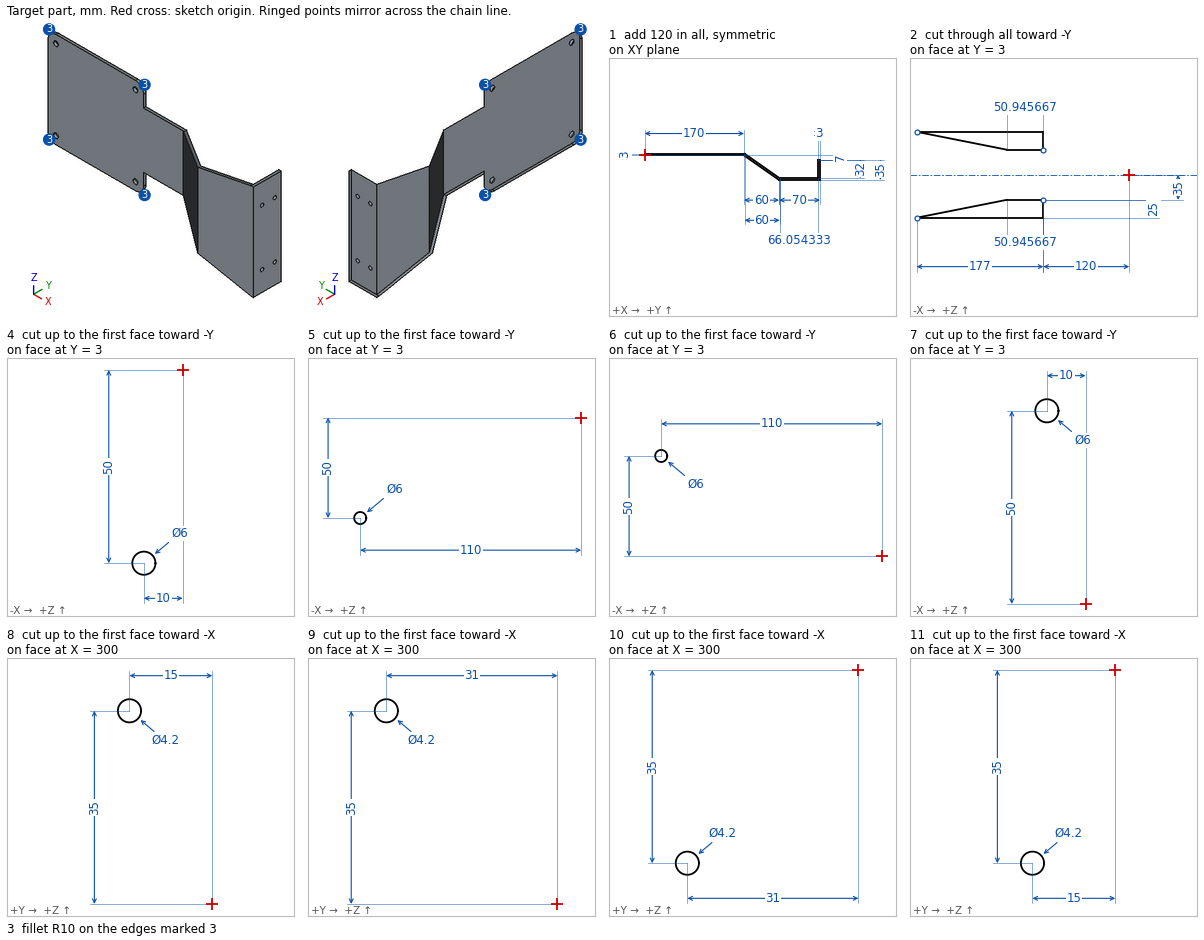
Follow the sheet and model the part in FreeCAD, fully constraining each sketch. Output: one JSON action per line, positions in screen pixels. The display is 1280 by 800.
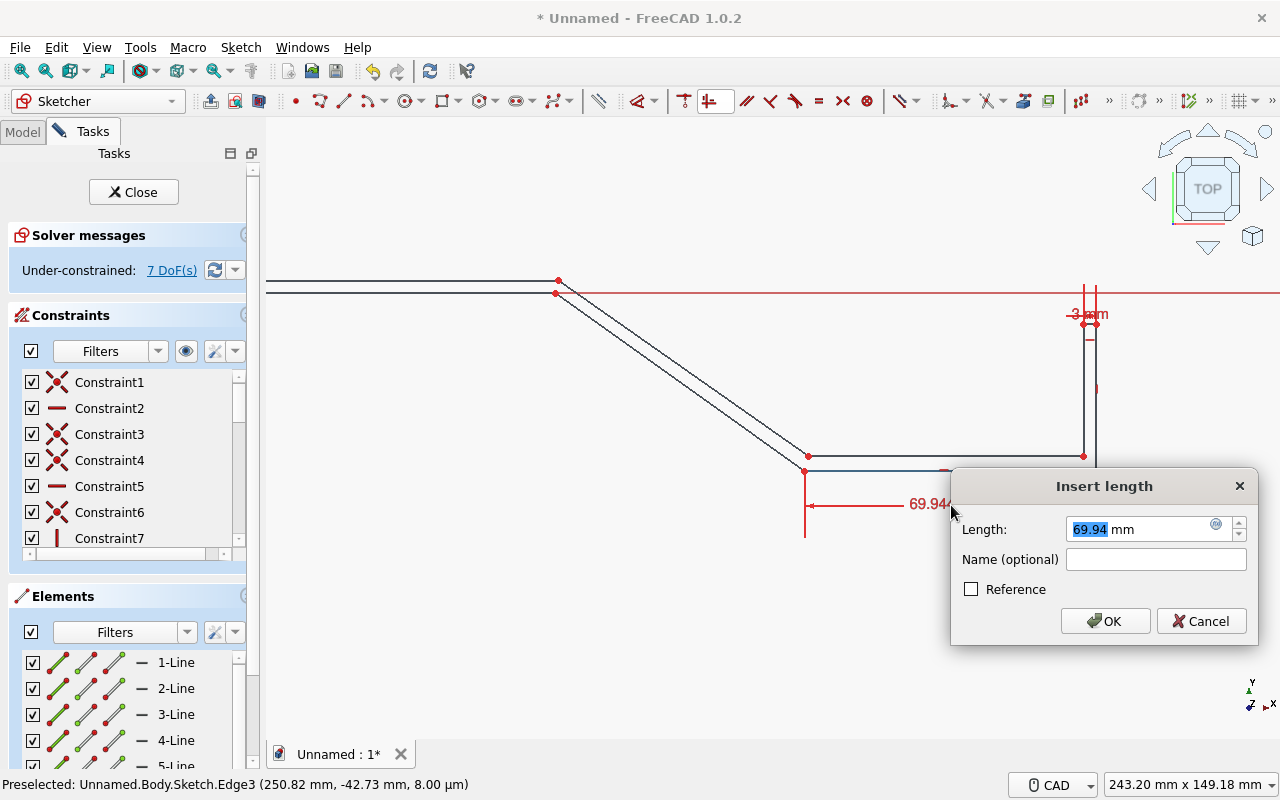
{"action": "type", "text": "70"}
{"action": "key", "text": "Return"}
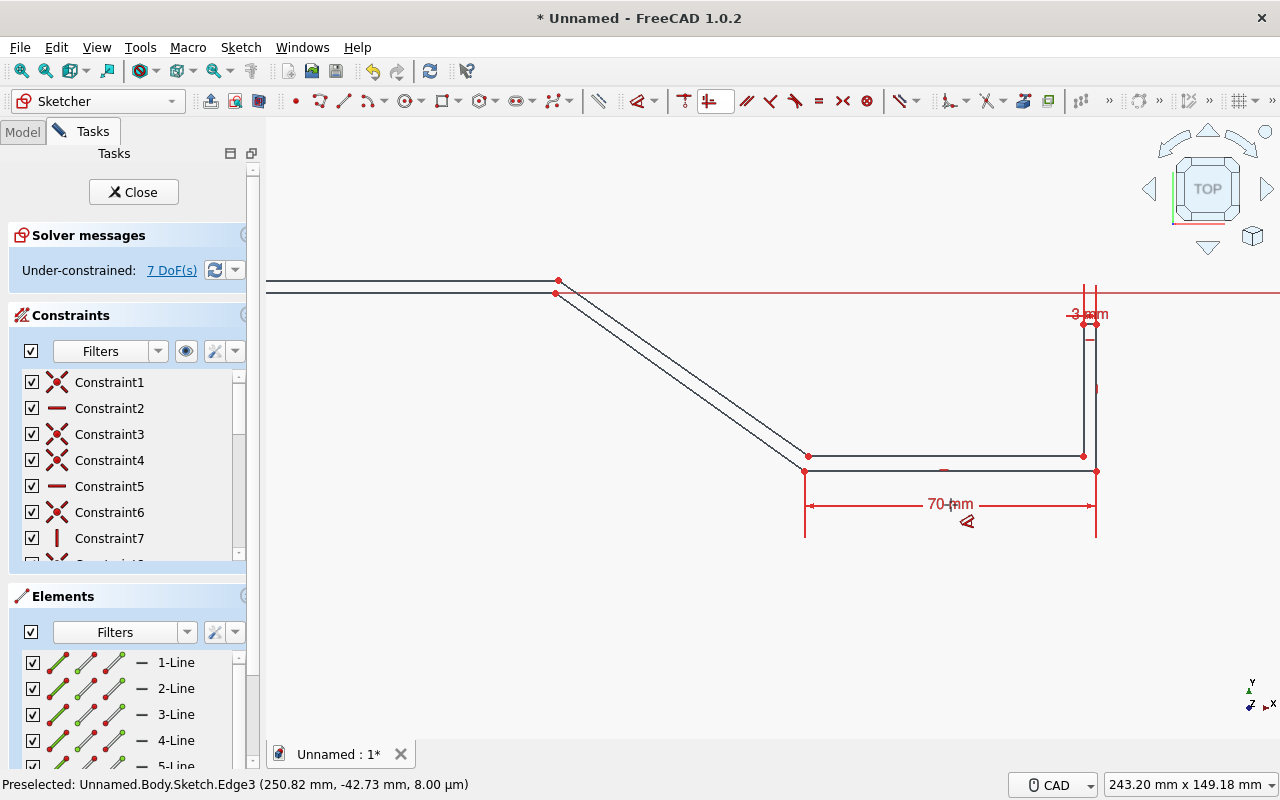
{"action": "left_click", "coordinate": [1096, 427]}
{"action": "left_click", "coordinate": [1062, 398]}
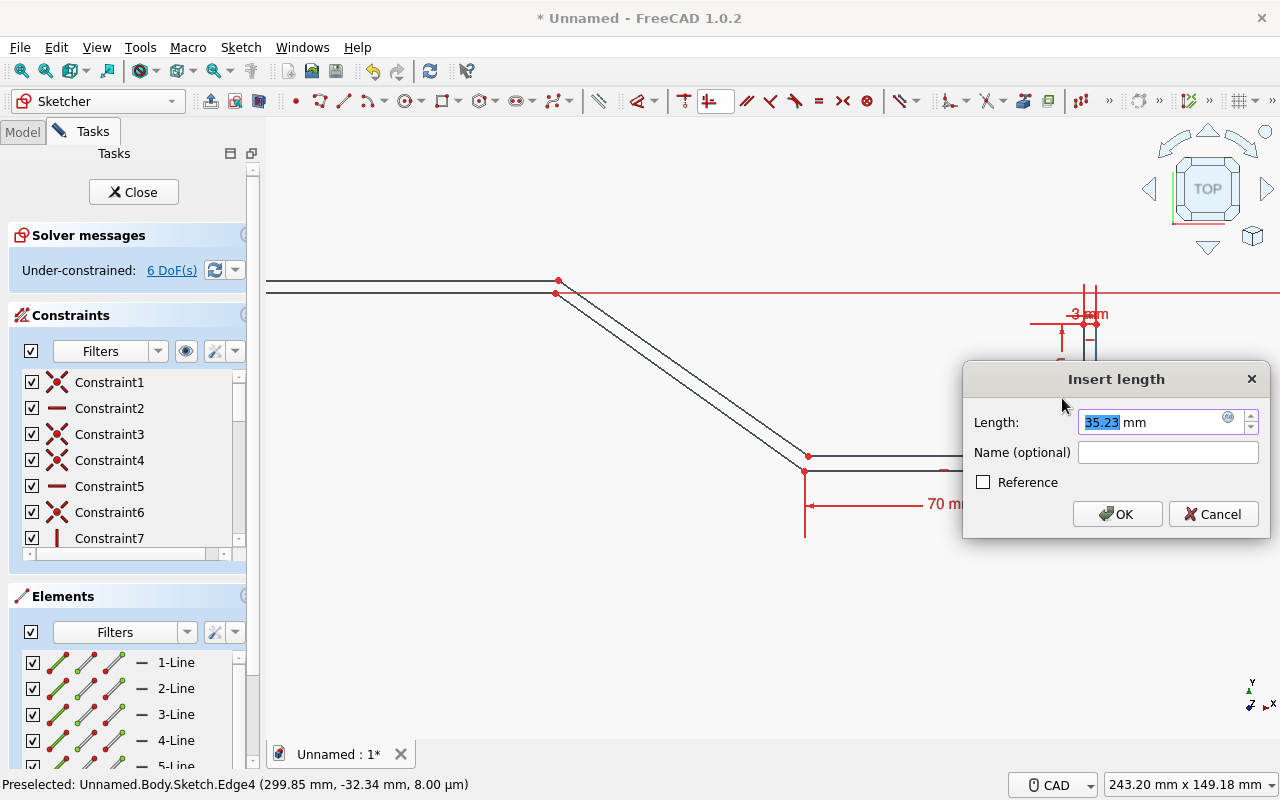
{"action": "type", "text": "35"}
{"action": "key", "text": "Return"}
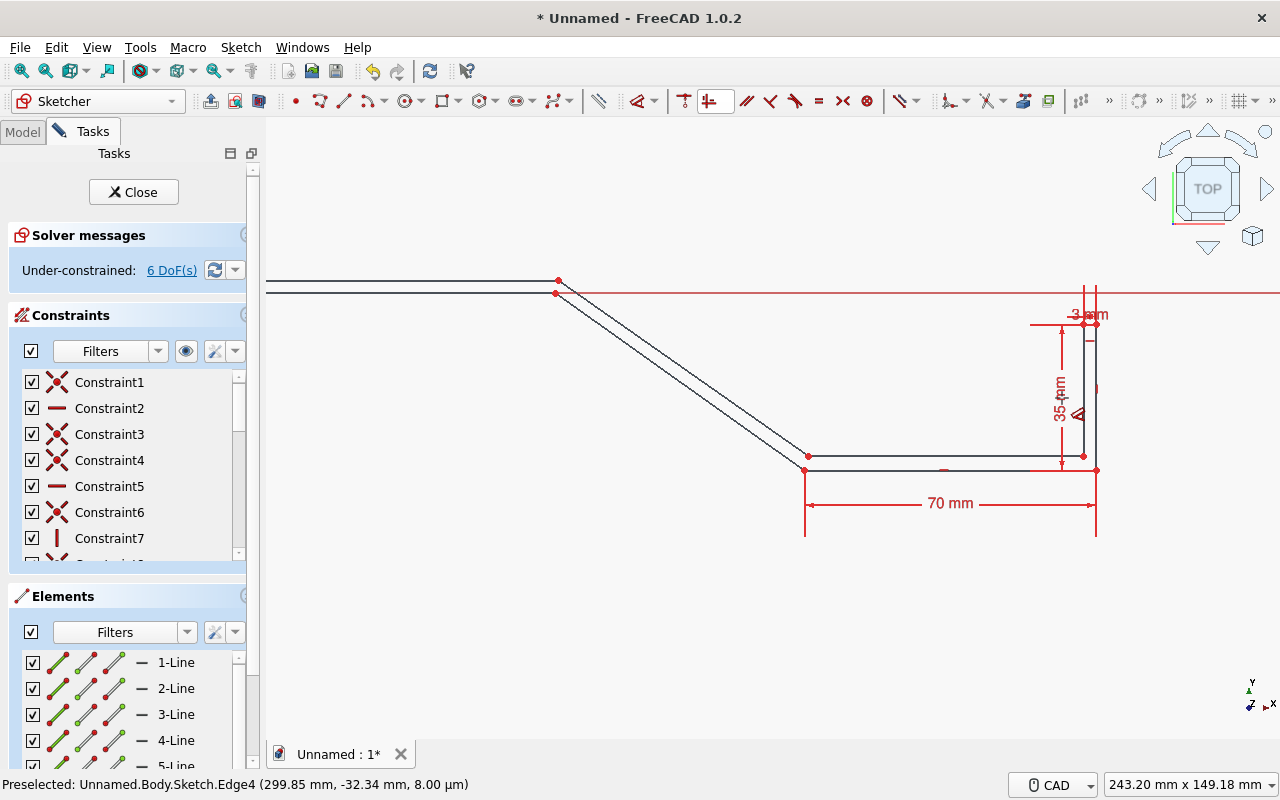
{"action": "left_click", "coordinate": [1084, 364]}
{"action": "left_click", "coordinate": [1050, 360]}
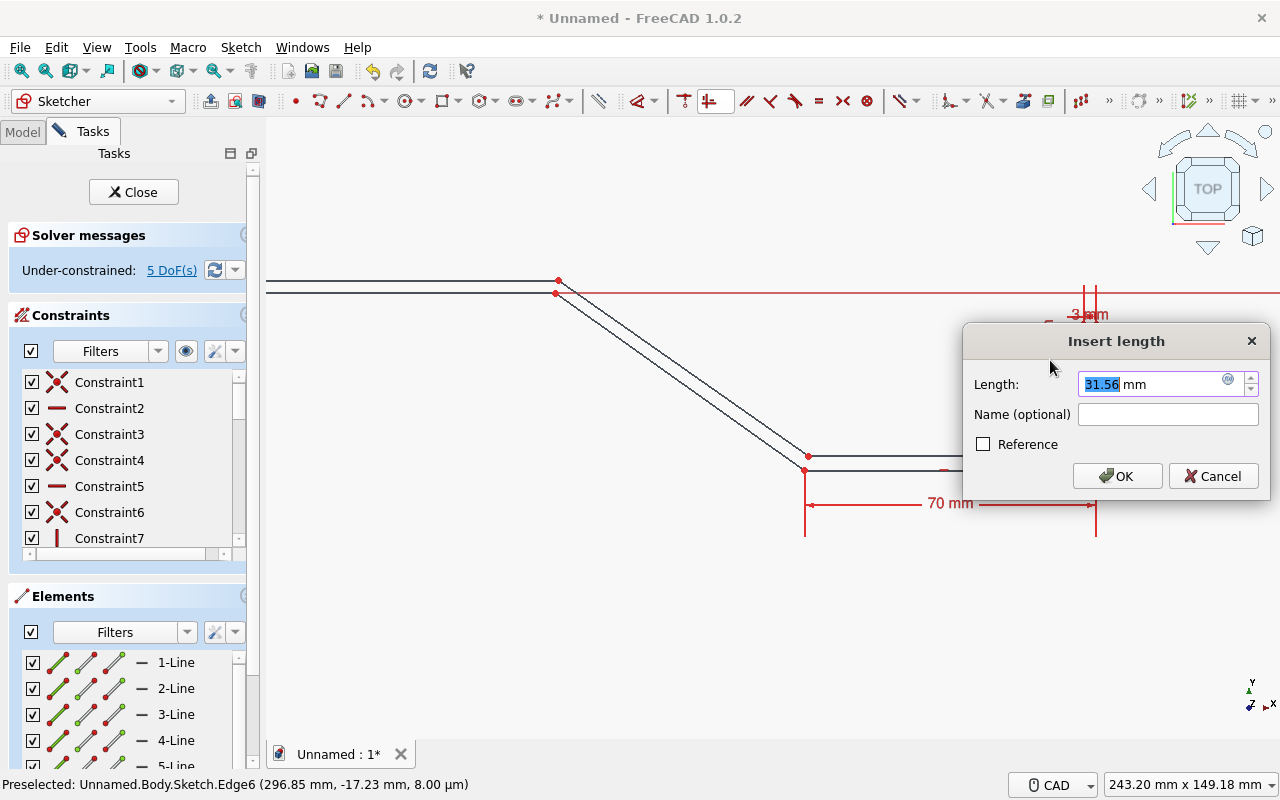
{"action": "type", "text": "32"}
{"action": "key", "text": "Return"}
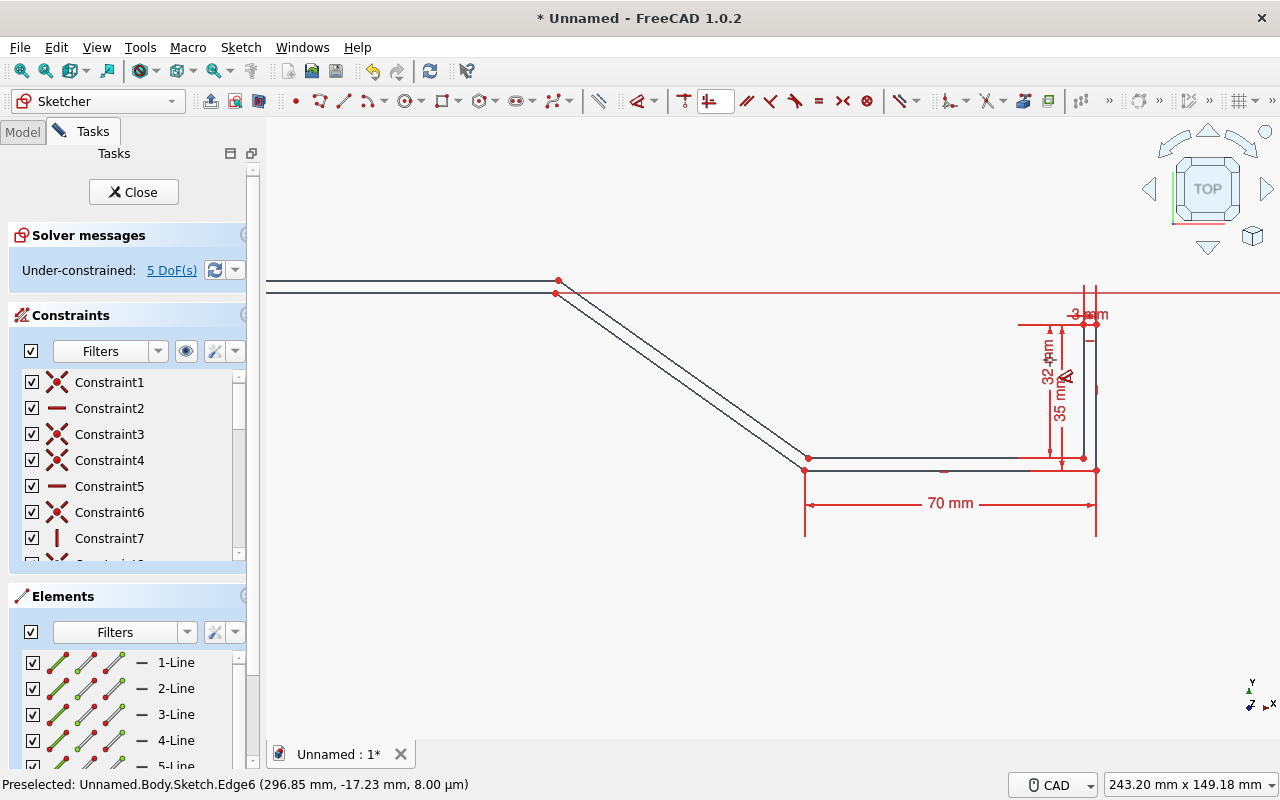
{"action": "scroll", "coordinate": [1096, 325], "scroll_direction": "up", "scroll_amount": 2}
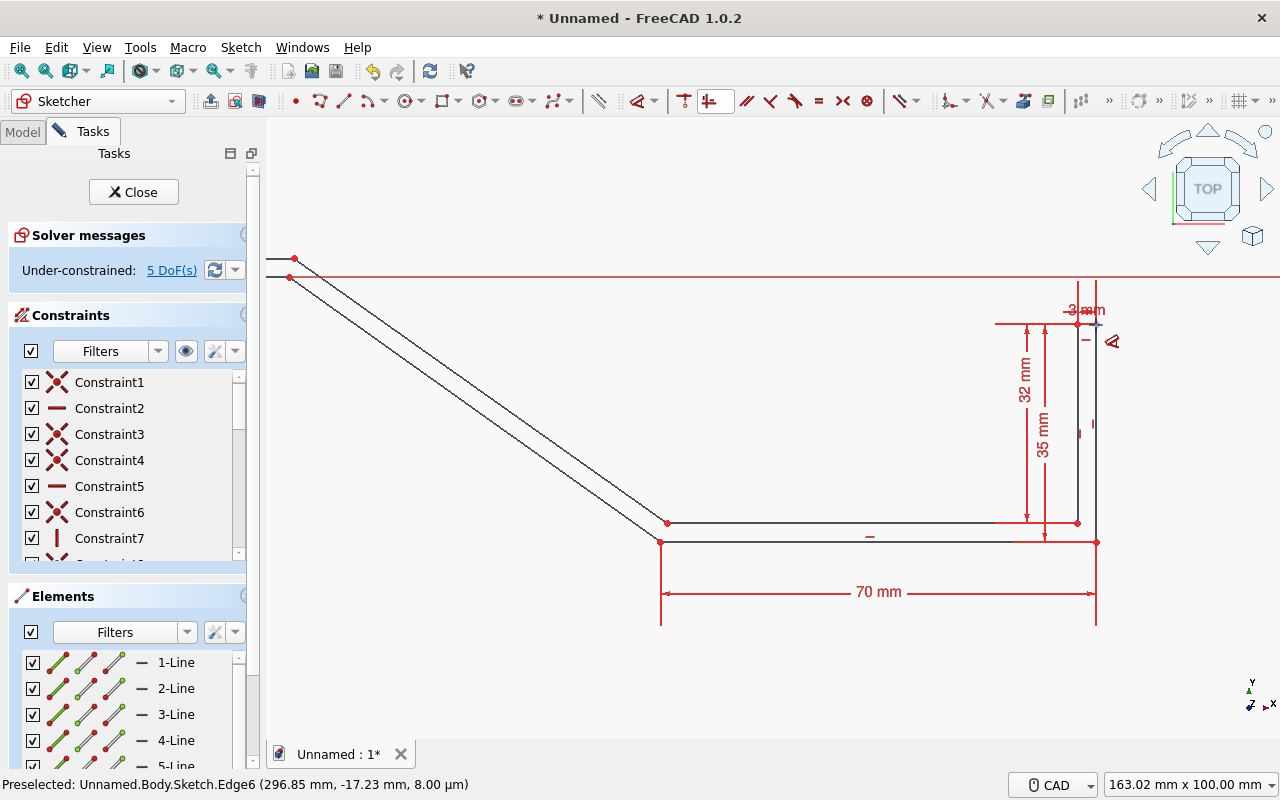
{"action": "left_click", "coordinate": [1096, 324]}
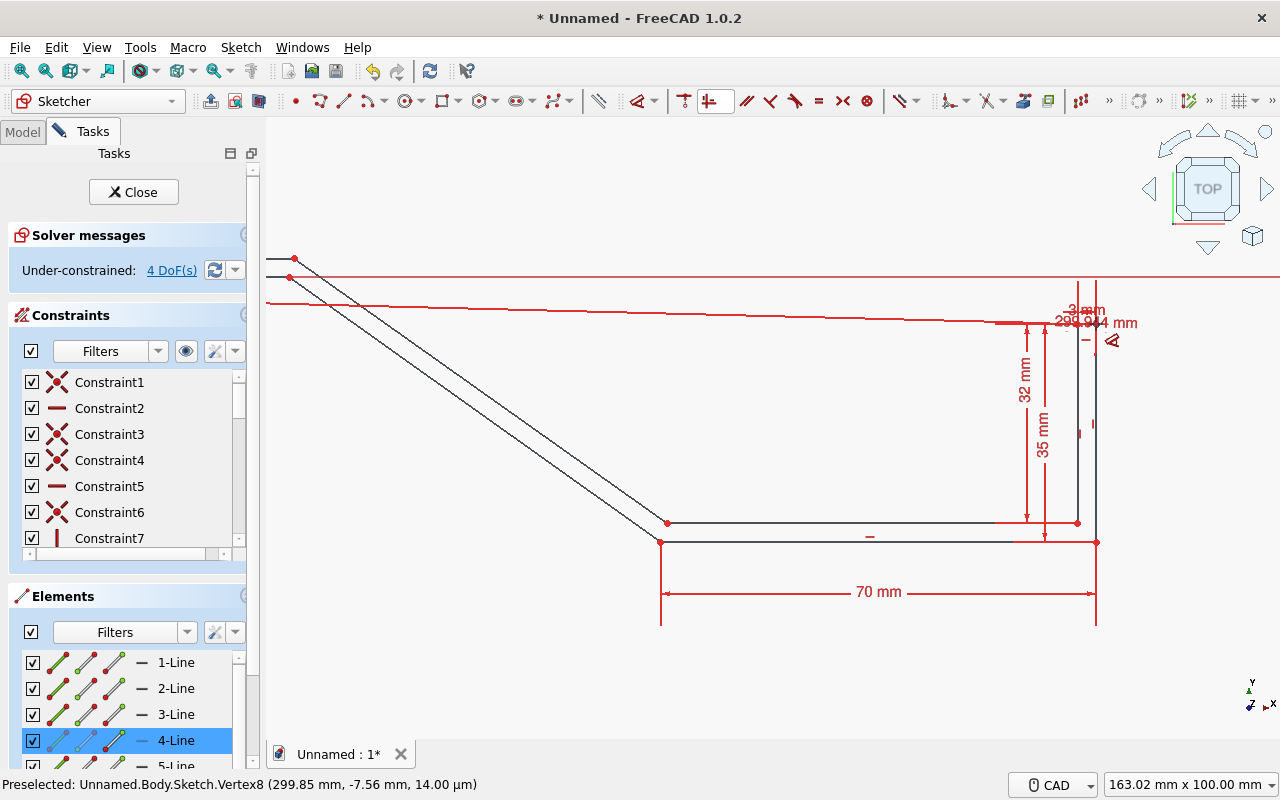
{"action": "key", "text": "Escape"}
{"action": "key", "text": "Escape"}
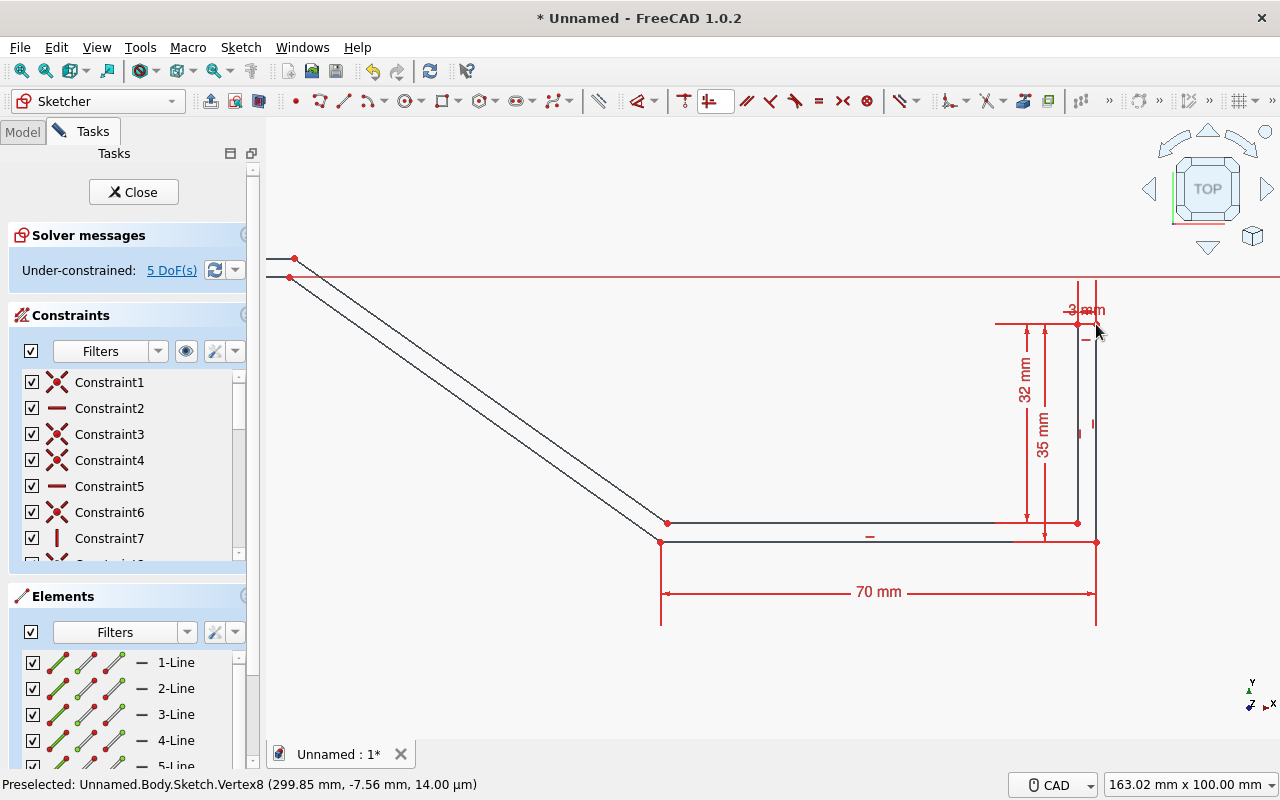
{"action": "left_click", "coordinate": [1096, 324]}